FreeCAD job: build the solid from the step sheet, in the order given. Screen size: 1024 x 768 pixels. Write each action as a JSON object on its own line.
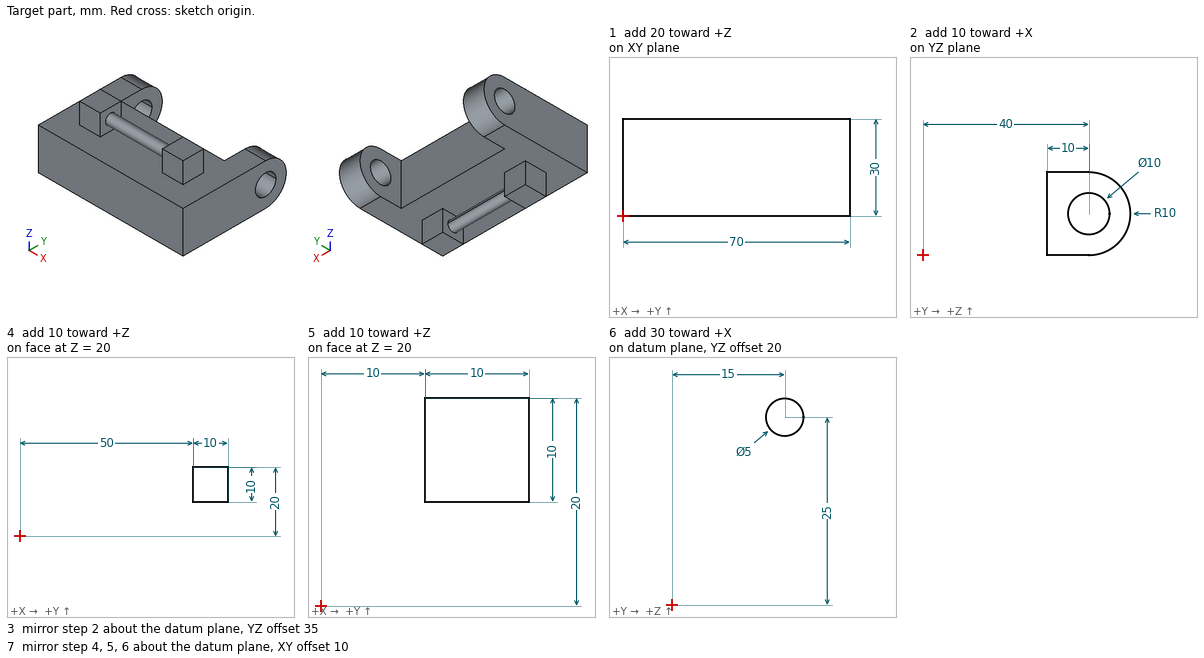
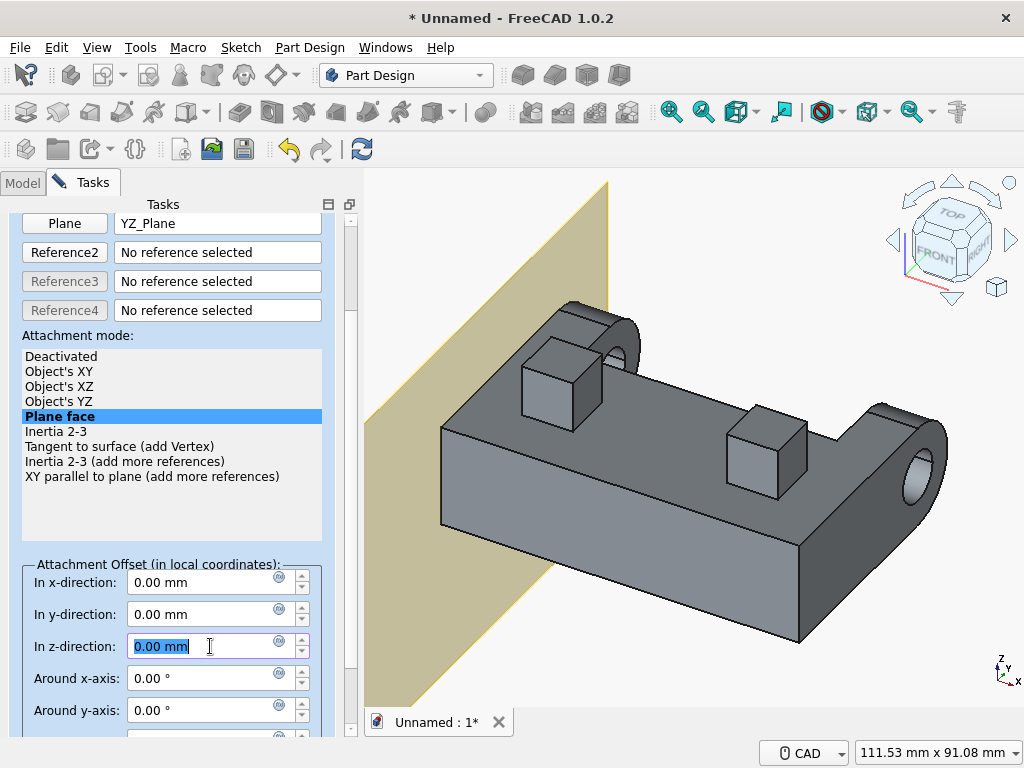
{"action": "type", "text": "20"}
{"action": "key", "text": "Tab"}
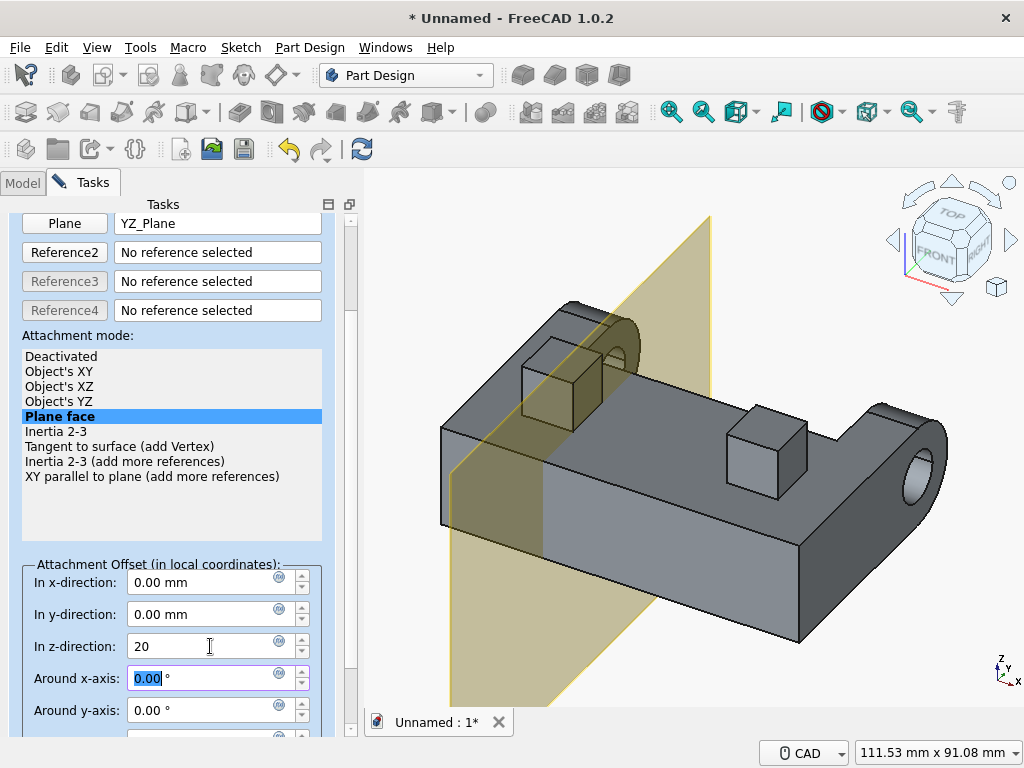
{"action": "scroll", "coordinate": [351, 475], "scroll_direction": "up", "scroll_amount": 3}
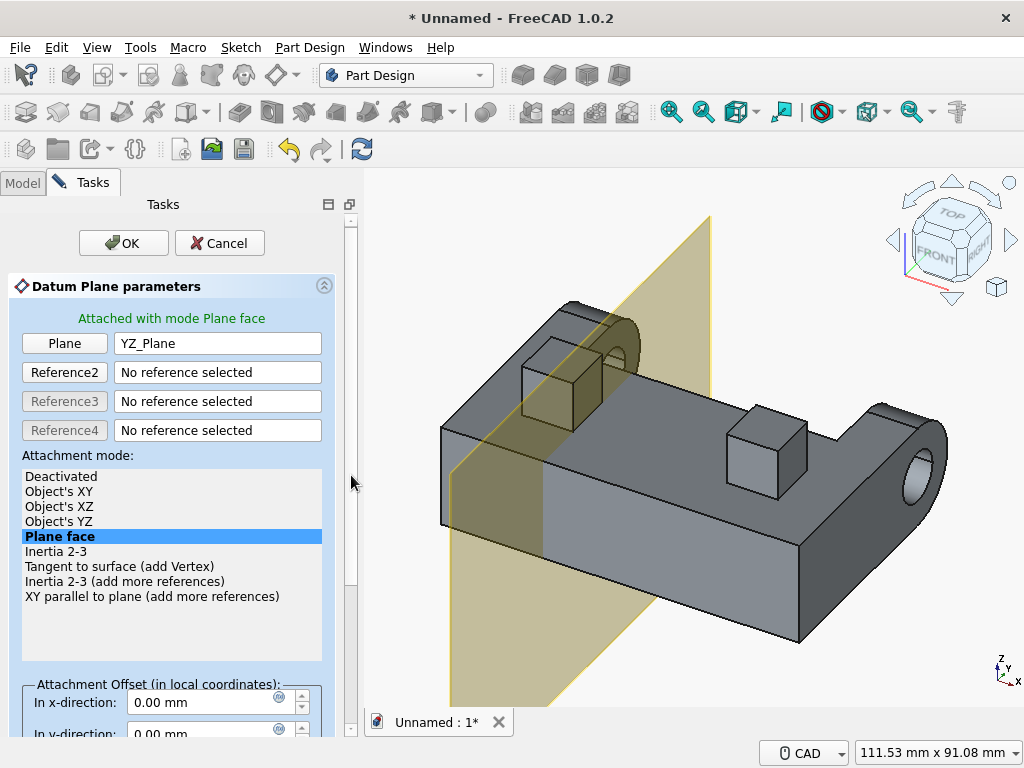
{"action": "left_click", "coordinate": [124, 243]}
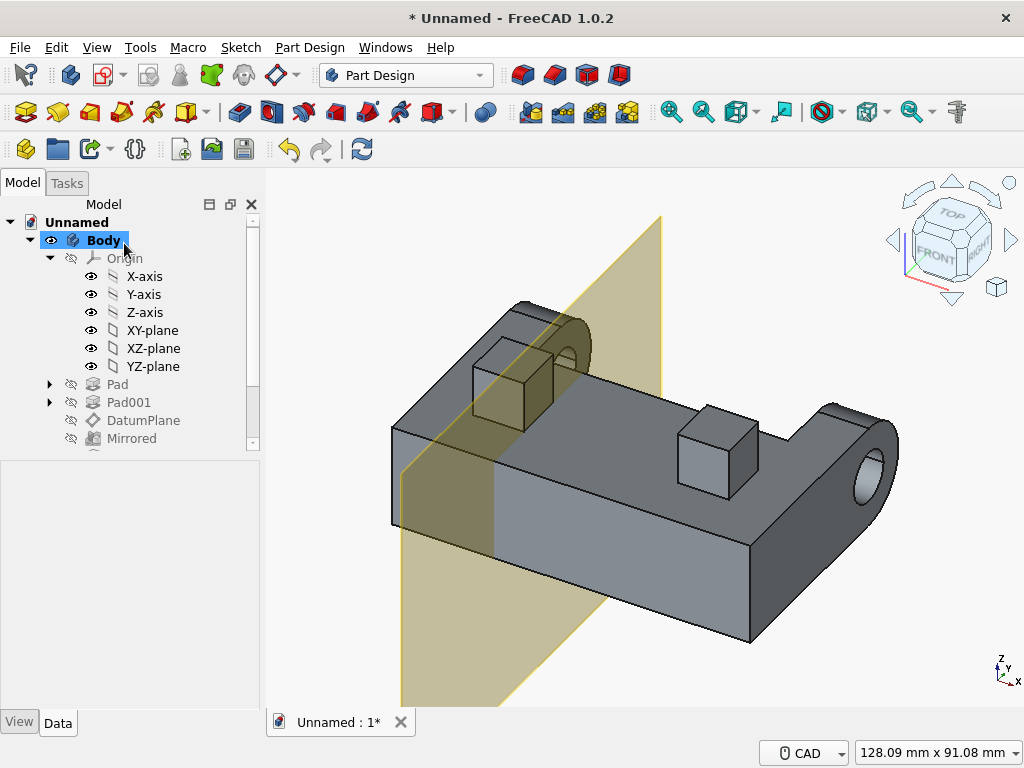
{"action": "scroll", "coordinate": [100, 326], "scroll_direction": "down", "scroll_amount": 3}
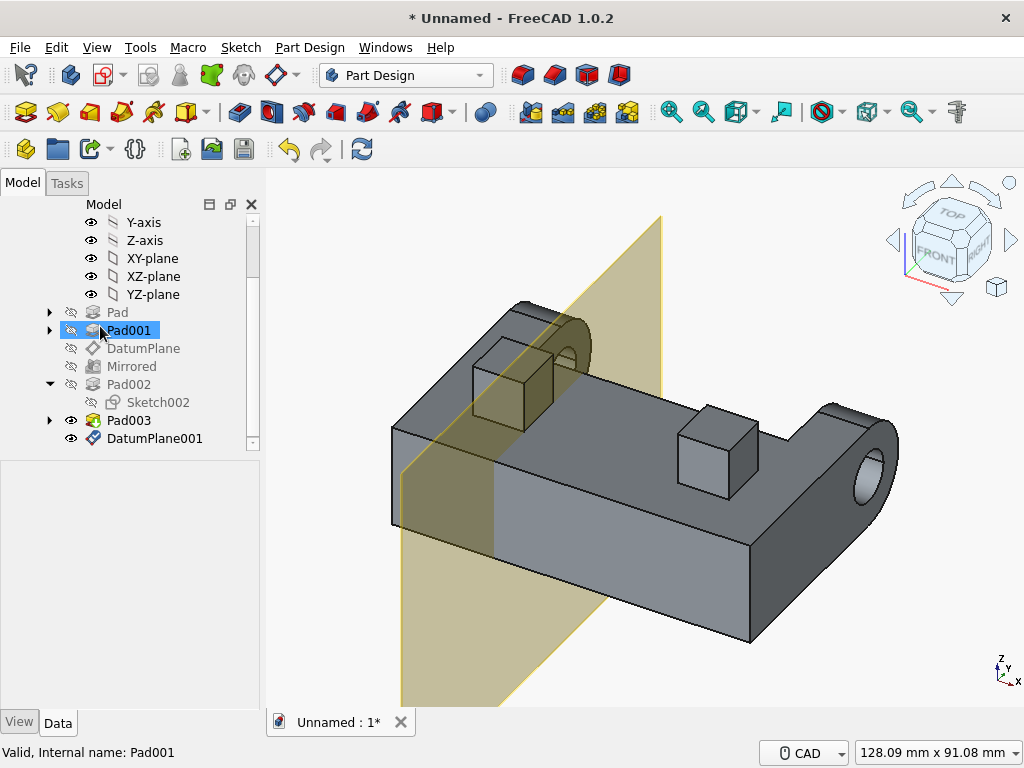
{"action": "left_click", "coordinate": [116, 438]}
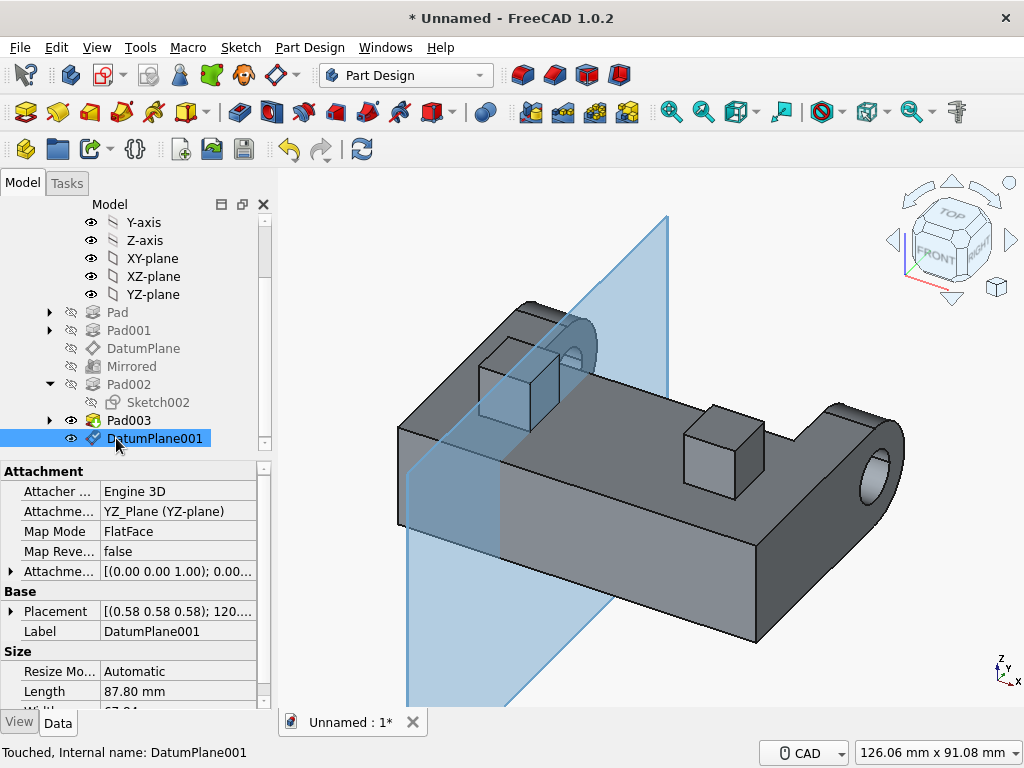
{"action": "left_click", "coordinate": [104, 76]}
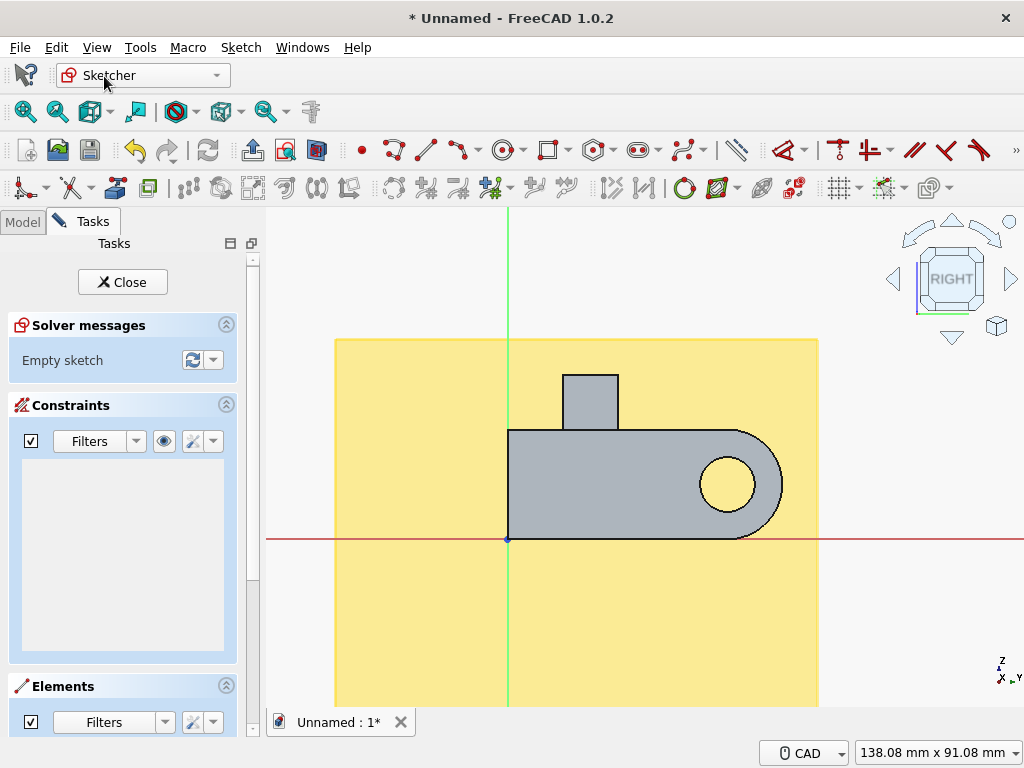
{"action": "key", "text": "q s"}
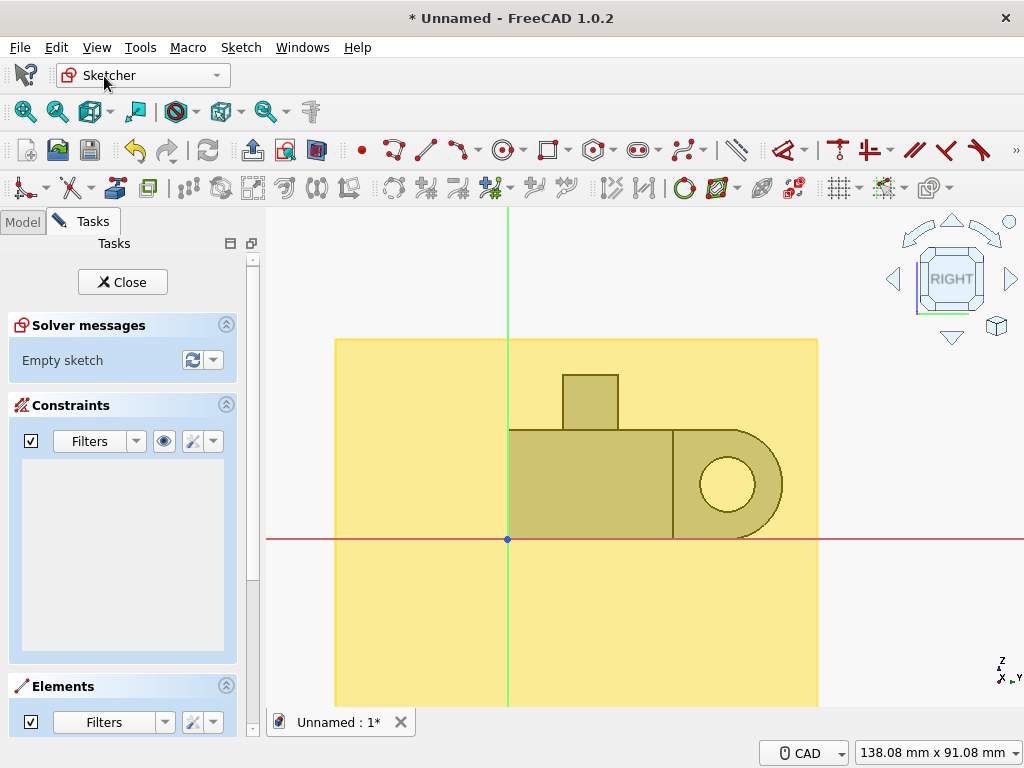
{"action": "scroll", "coordinate": [592, 397], "scroll_direction": "up", "scroll_amount": 12}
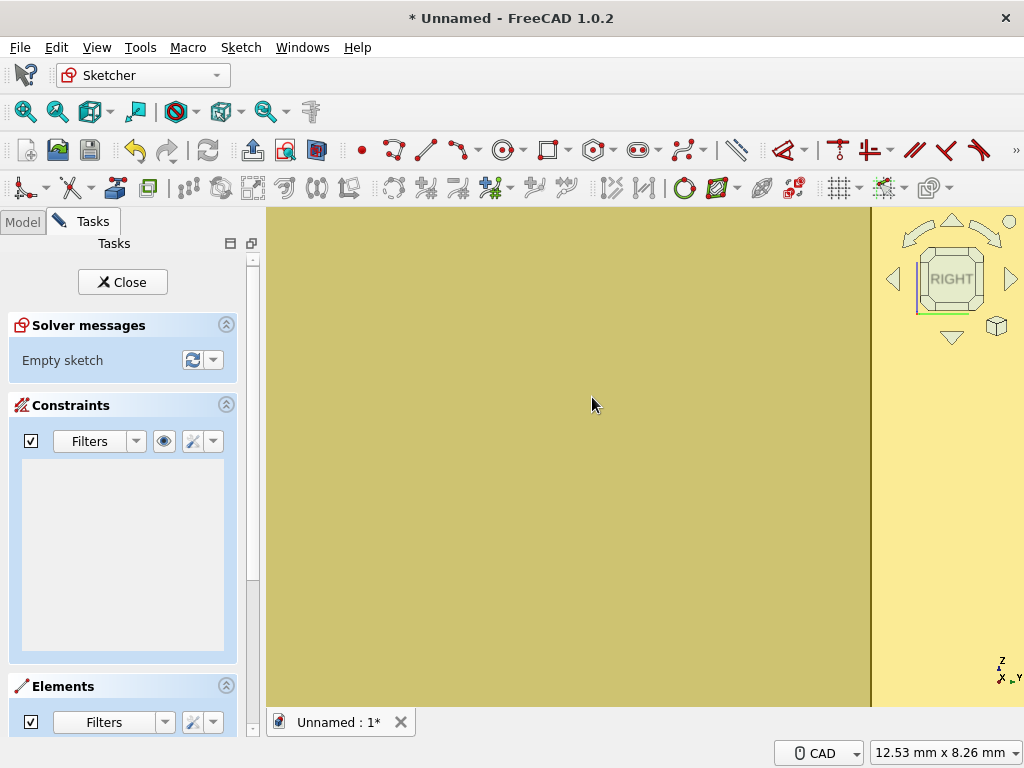
{"action": "left_click", "coordinate": [504, 150]}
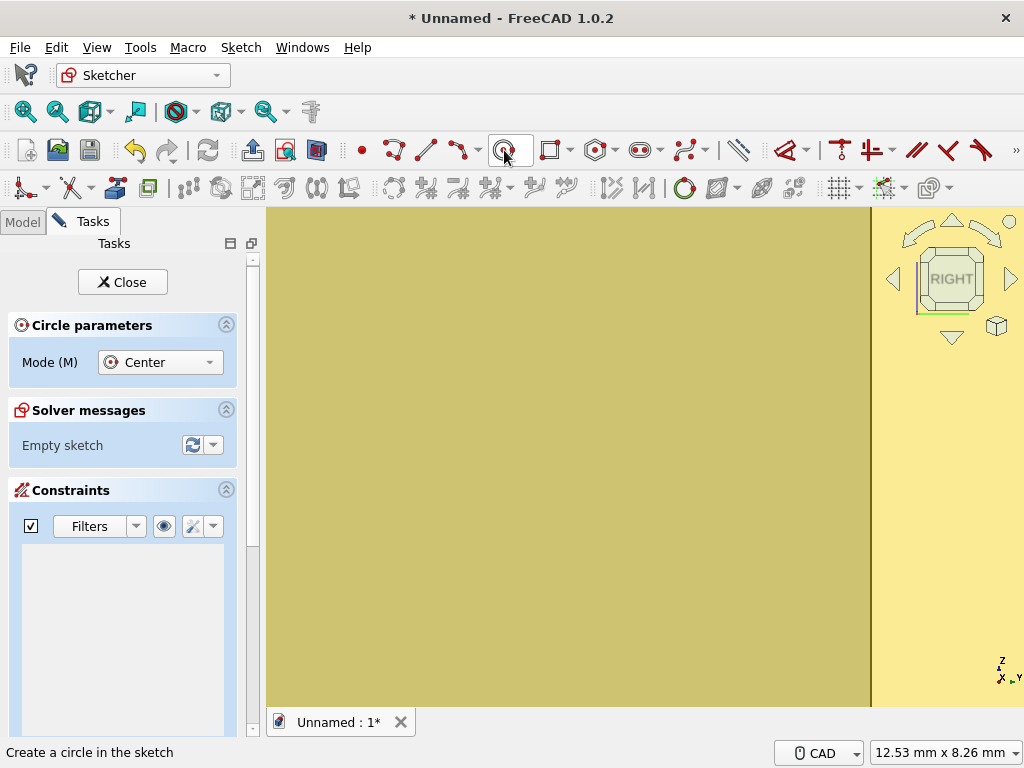
{"action": "left_click", "coordinate": [568, 449]}
{"action": "mouse_move", "coordinate": [675, 342]}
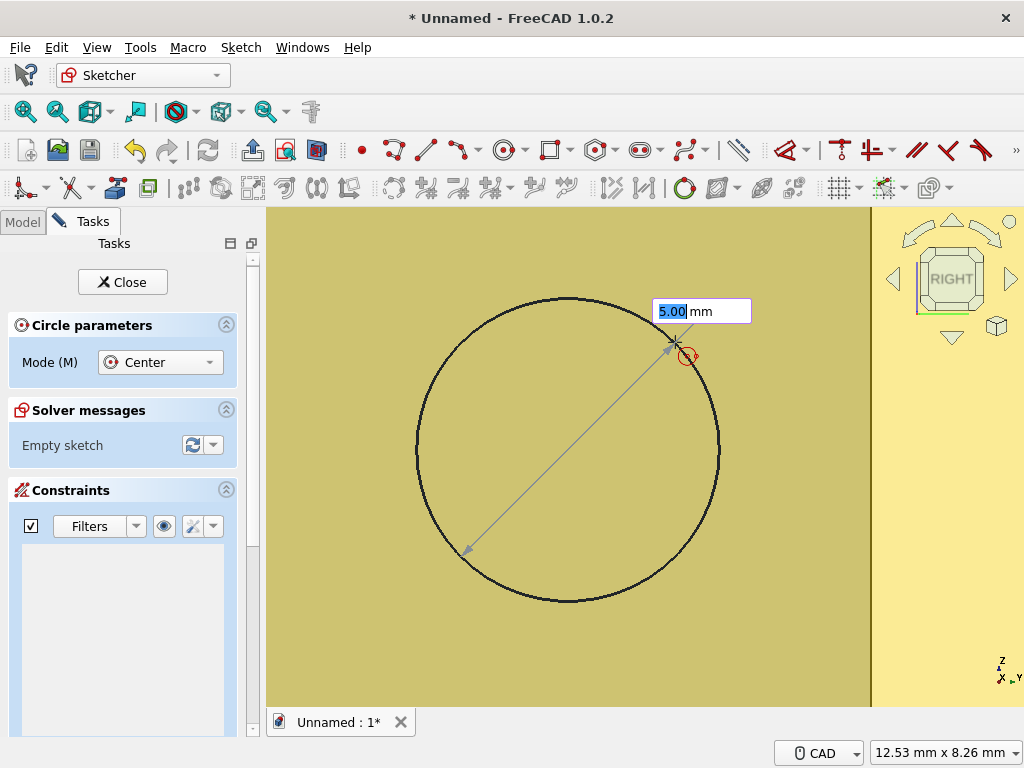
{"action": "type", "text": "5"}
{"action": "key", "text": "Return"}
{"action": "key", "text": "Escape"}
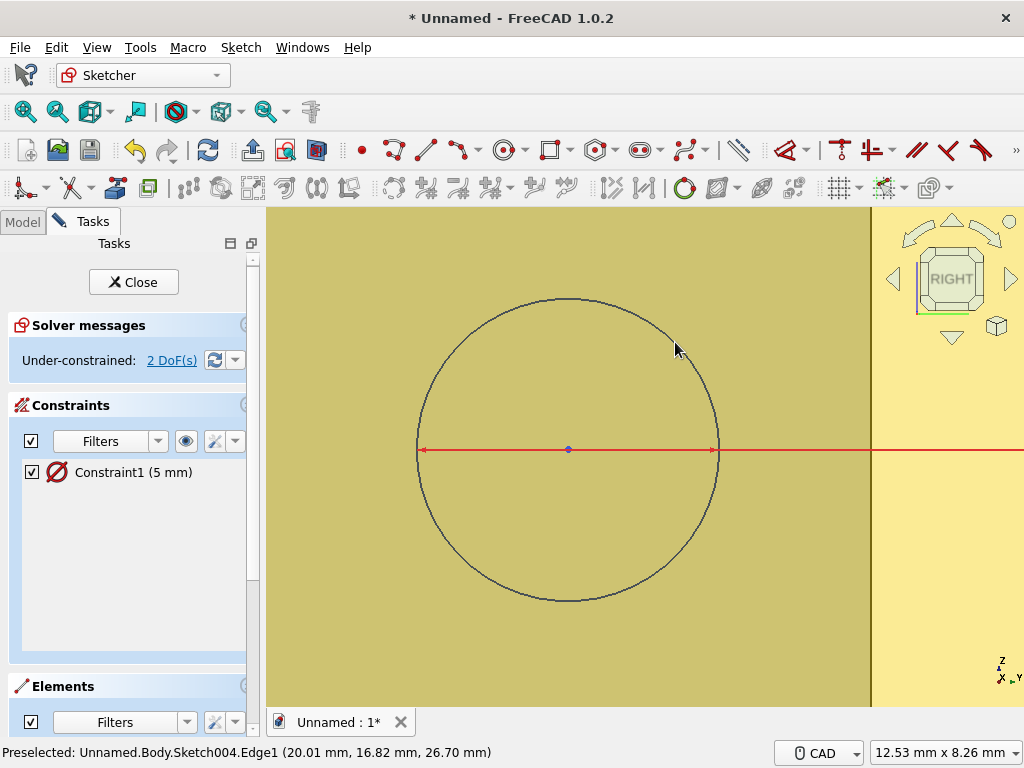
{"action": "key", "text": "d"}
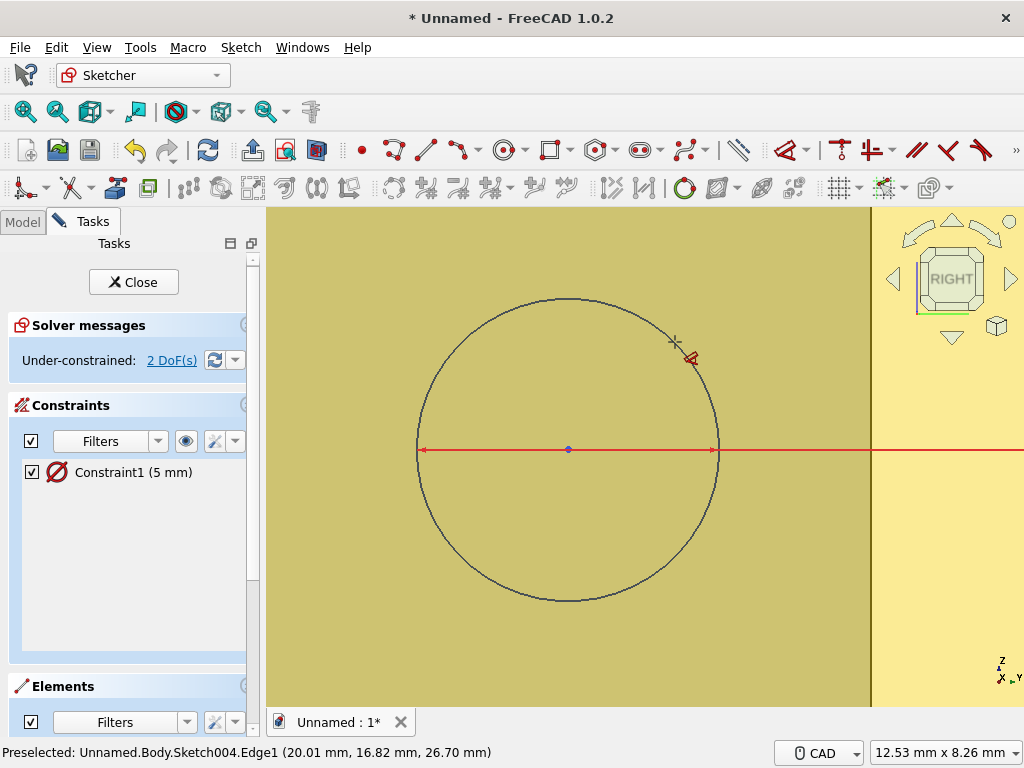
{"action": "left_click", "coordinate": [568, 450]}
{"action": "left_click", "coordinate": [368, 416]}